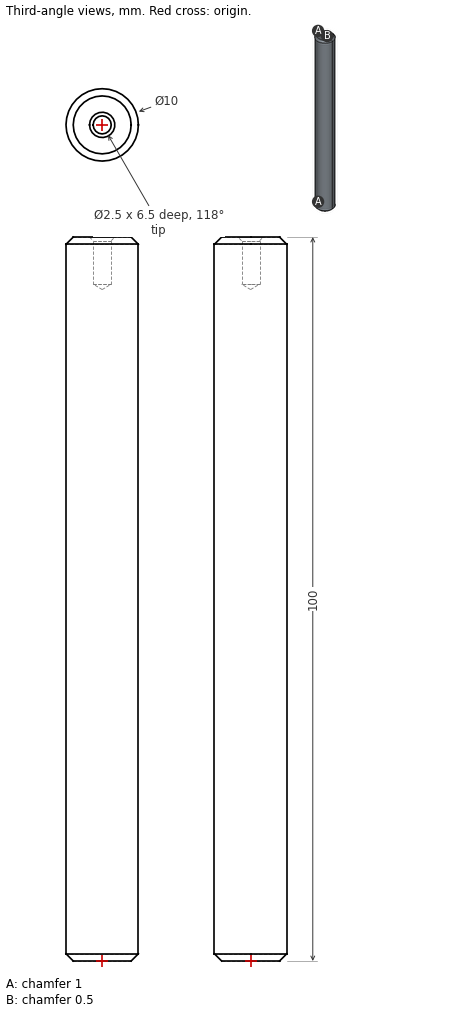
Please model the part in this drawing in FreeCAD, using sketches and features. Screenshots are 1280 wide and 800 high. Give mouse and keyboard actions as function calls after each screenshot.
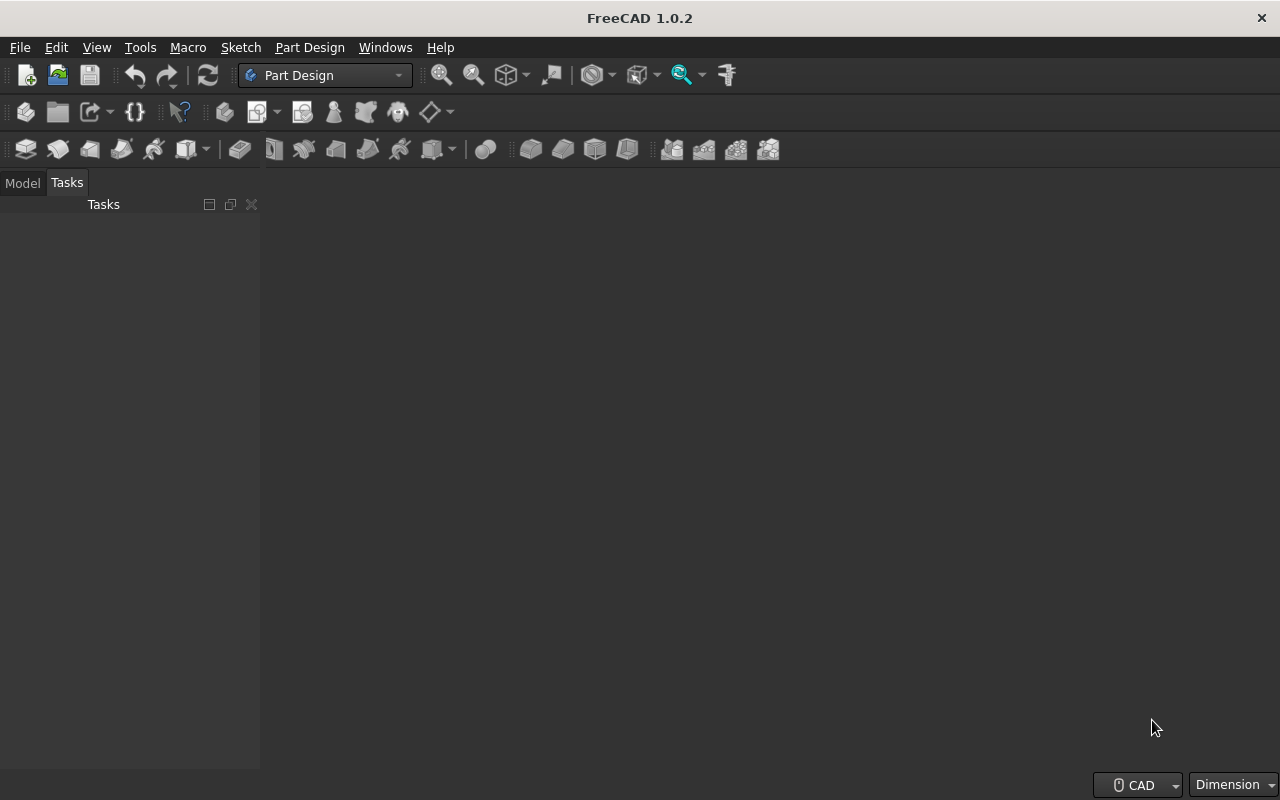
click(168, 112)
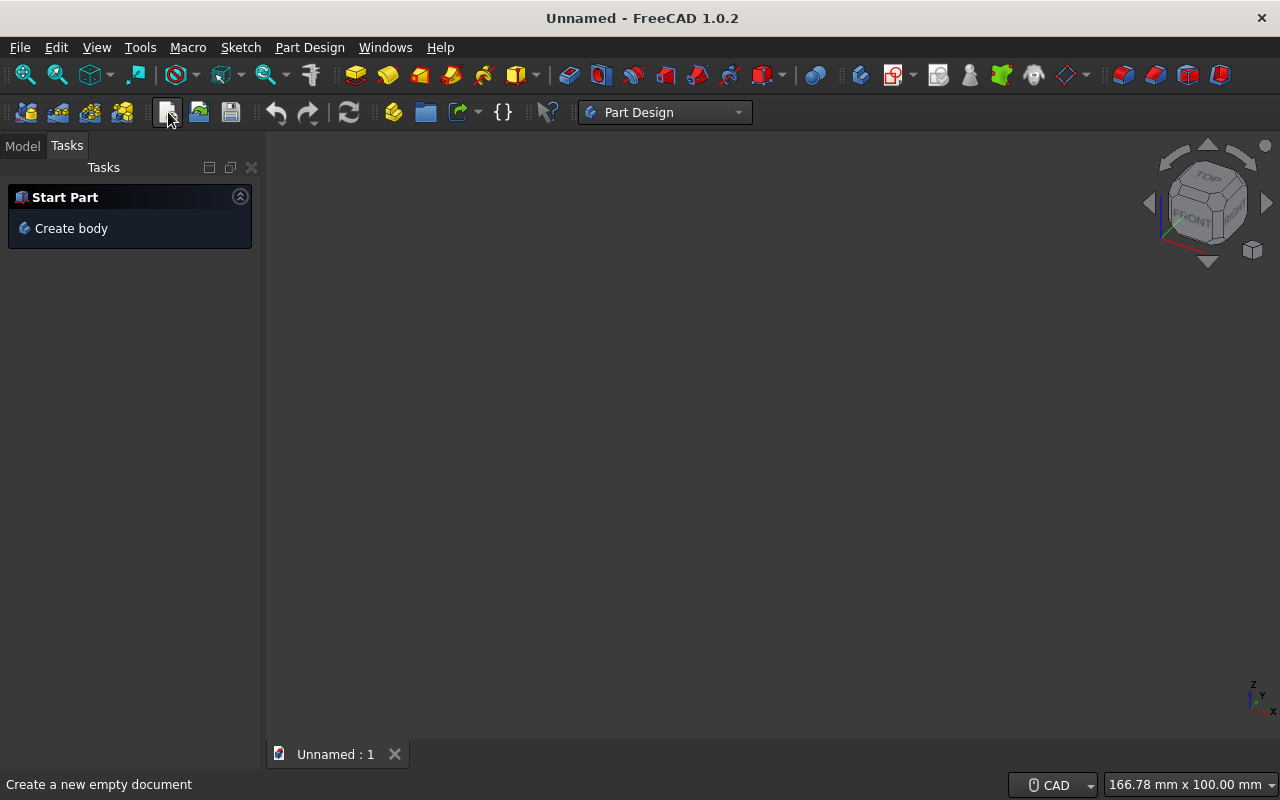
click(894, 76)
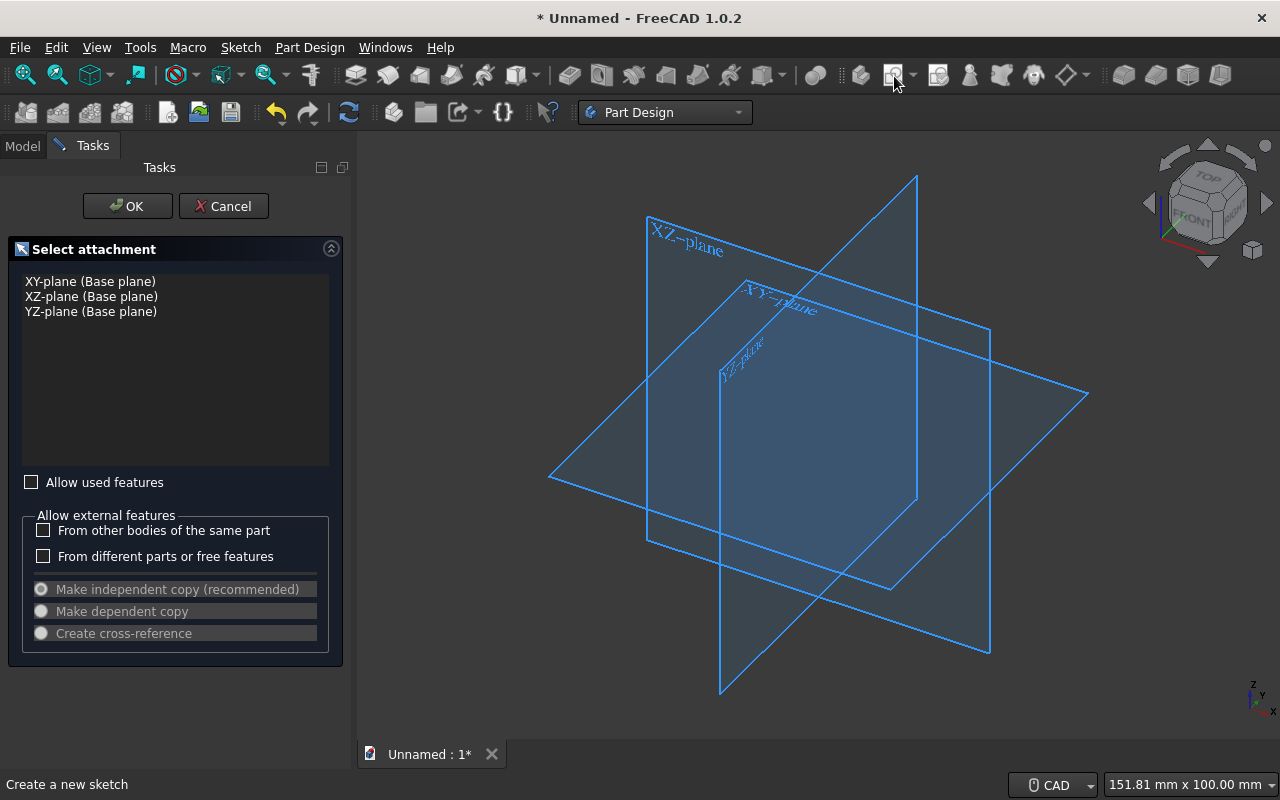
click(82, 282)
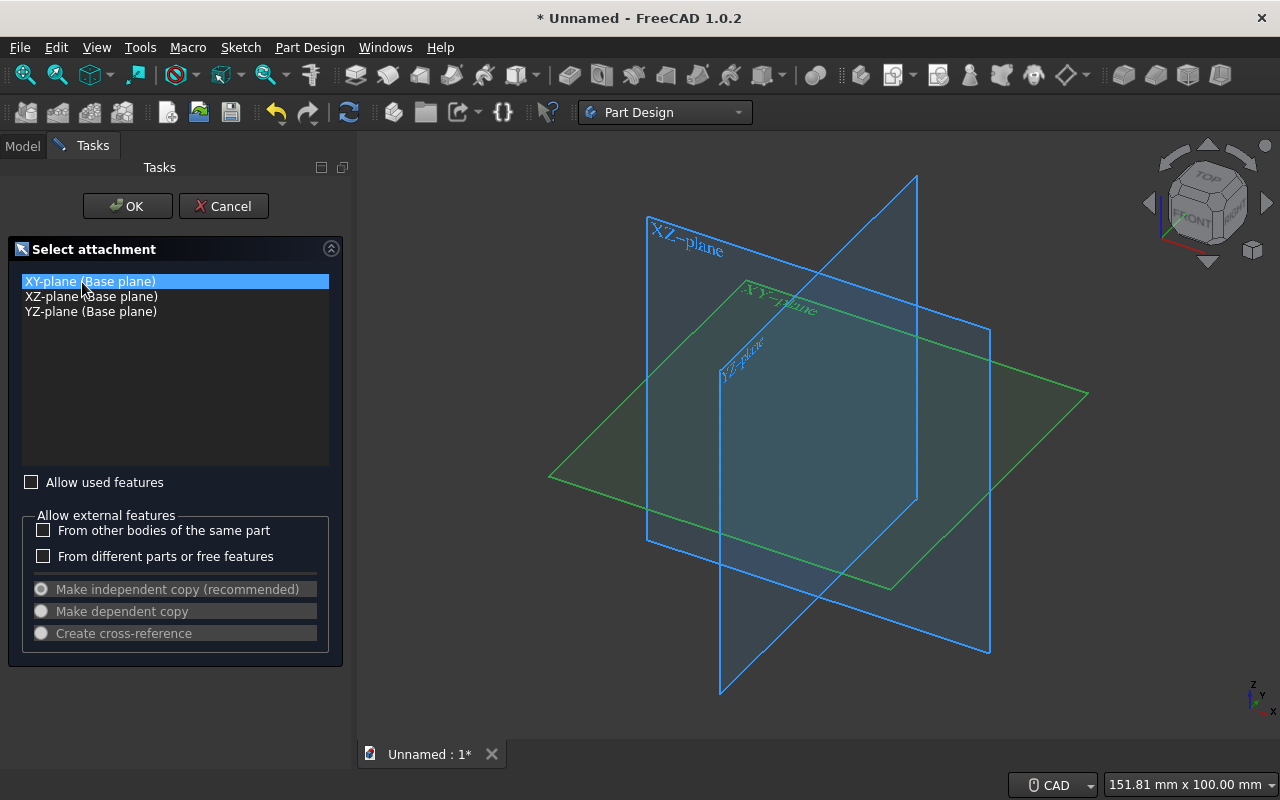
click(128, 206)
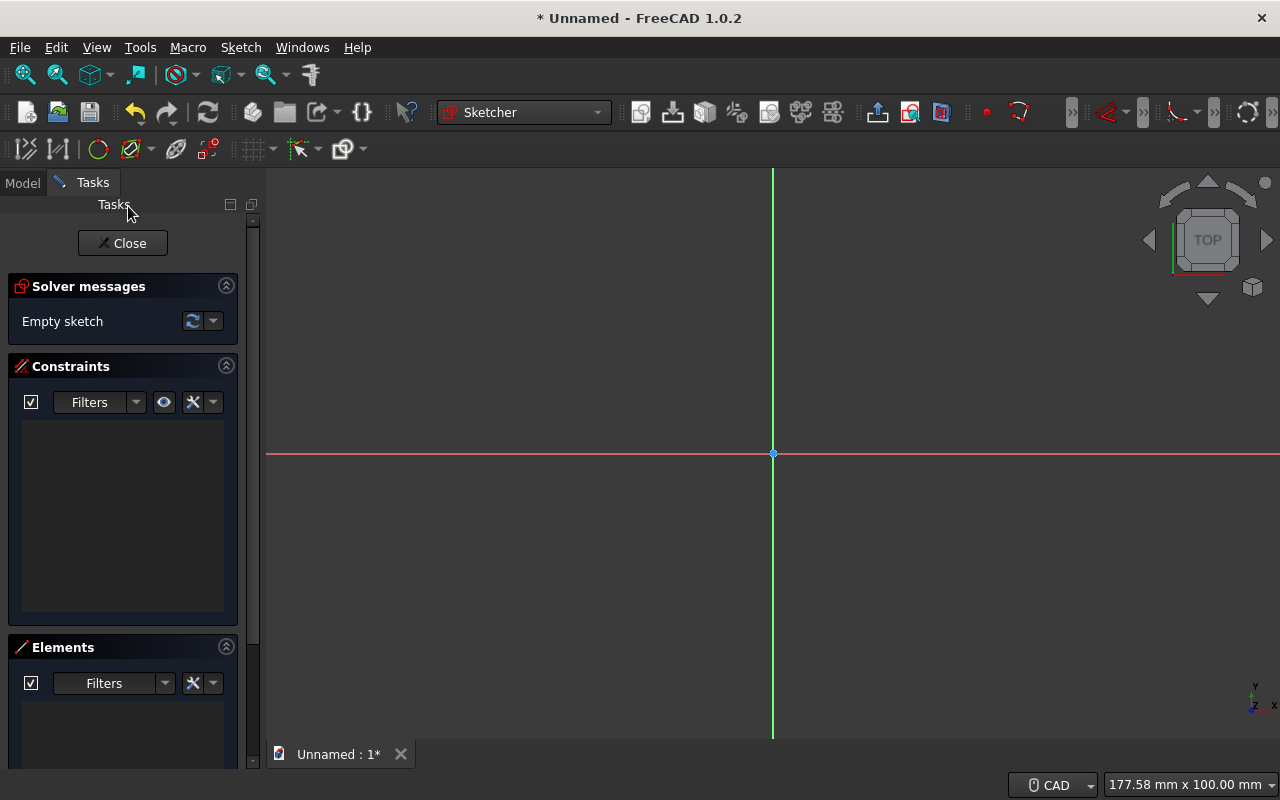
scroll(787, 454, up, 9)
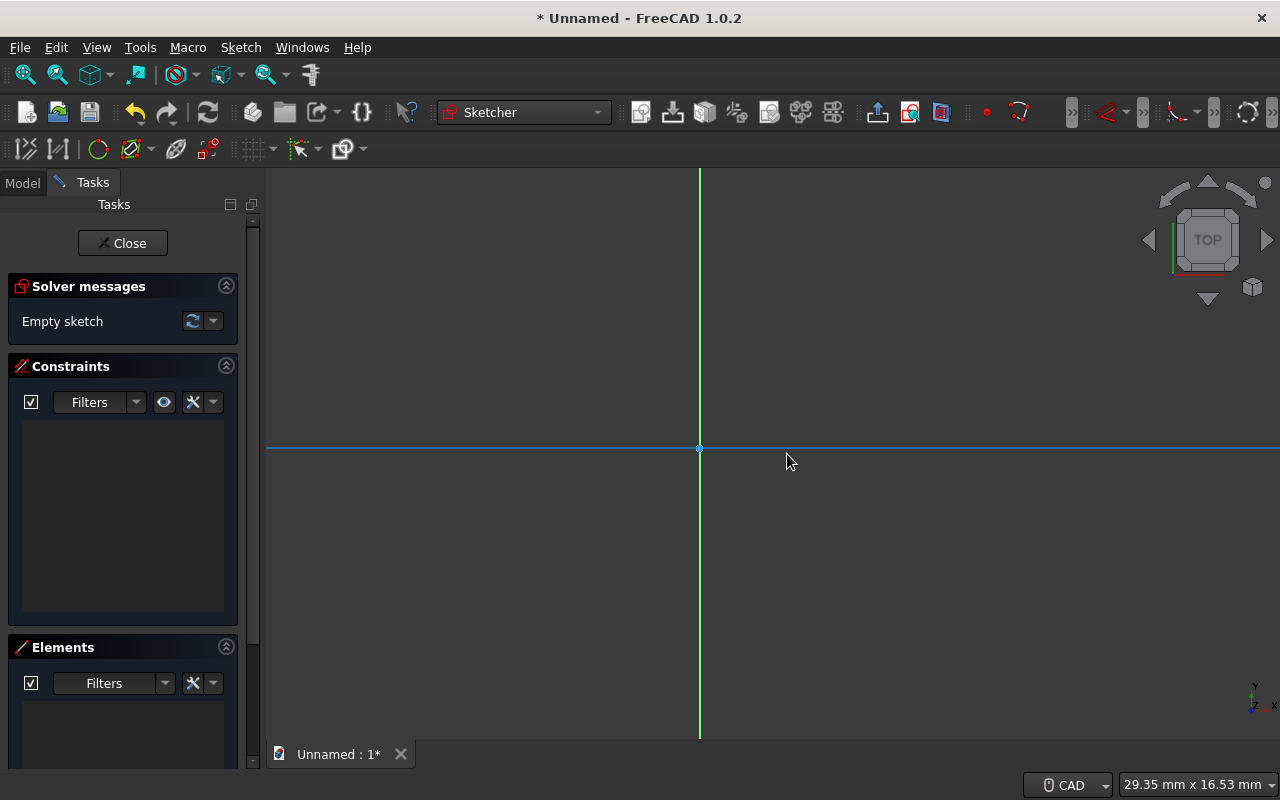
key(g)
key(c)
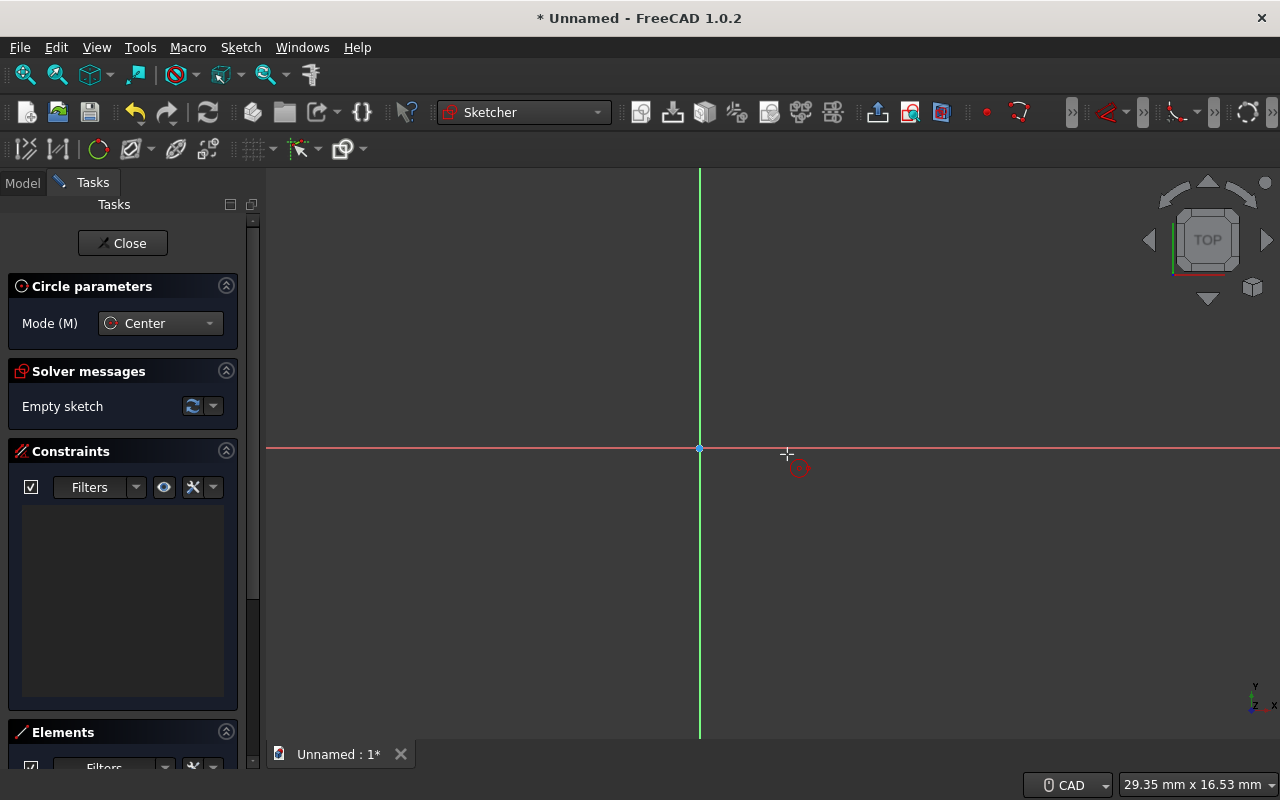
click(700, 448)
move(822, 326)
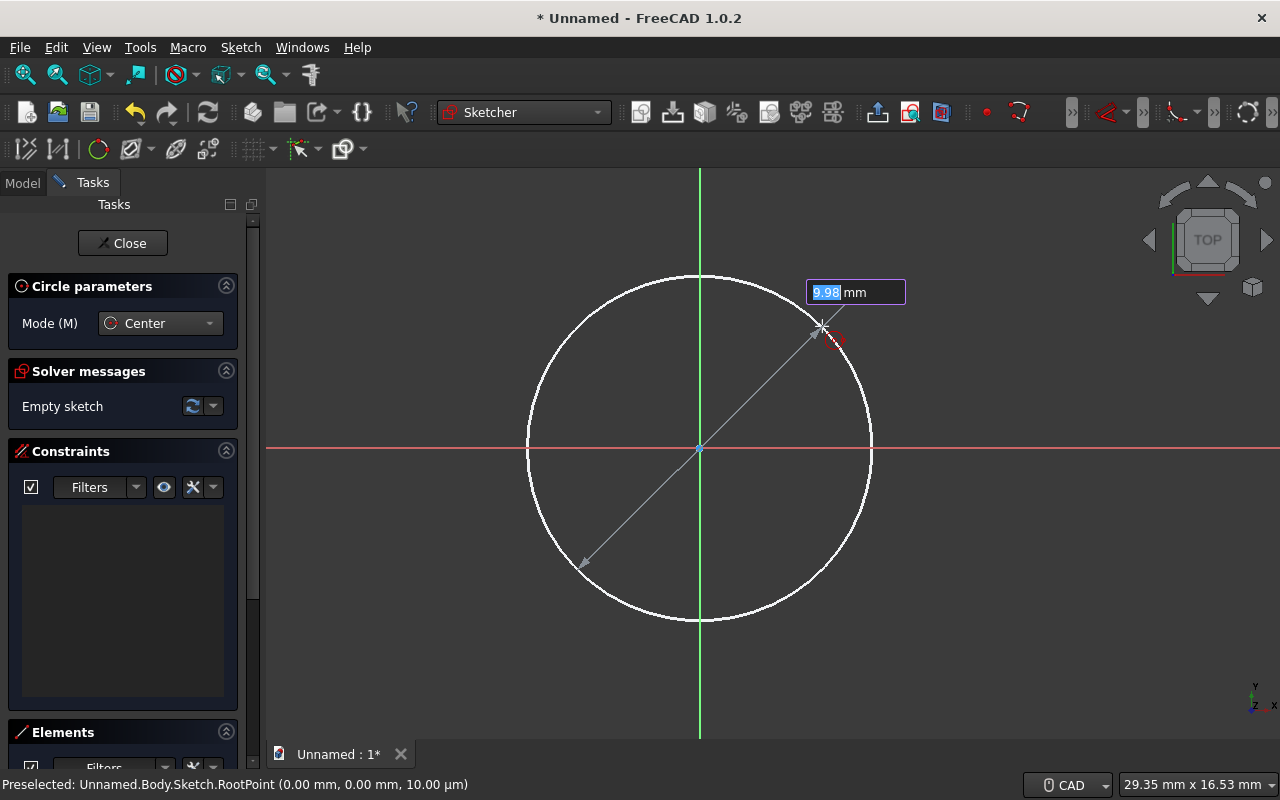
text(10)
key(Return)
key(Escape)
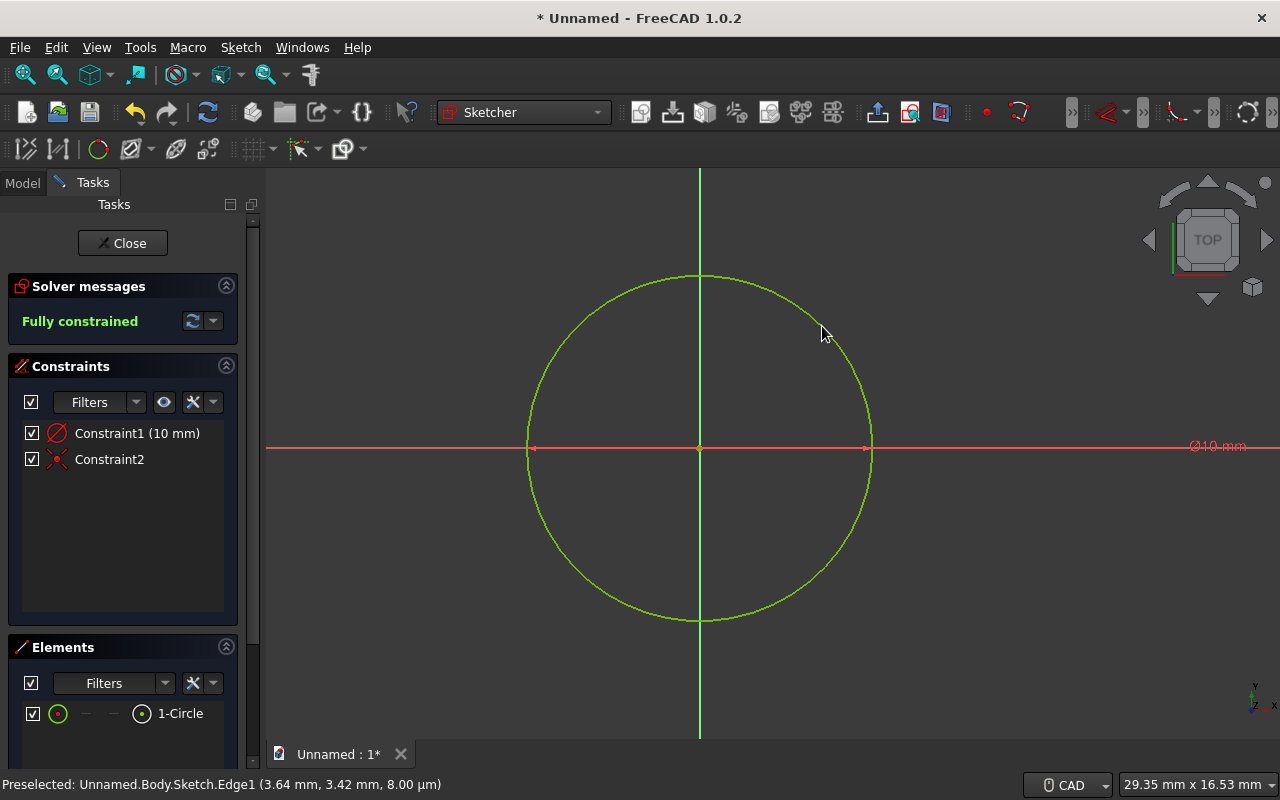
click(123, 243)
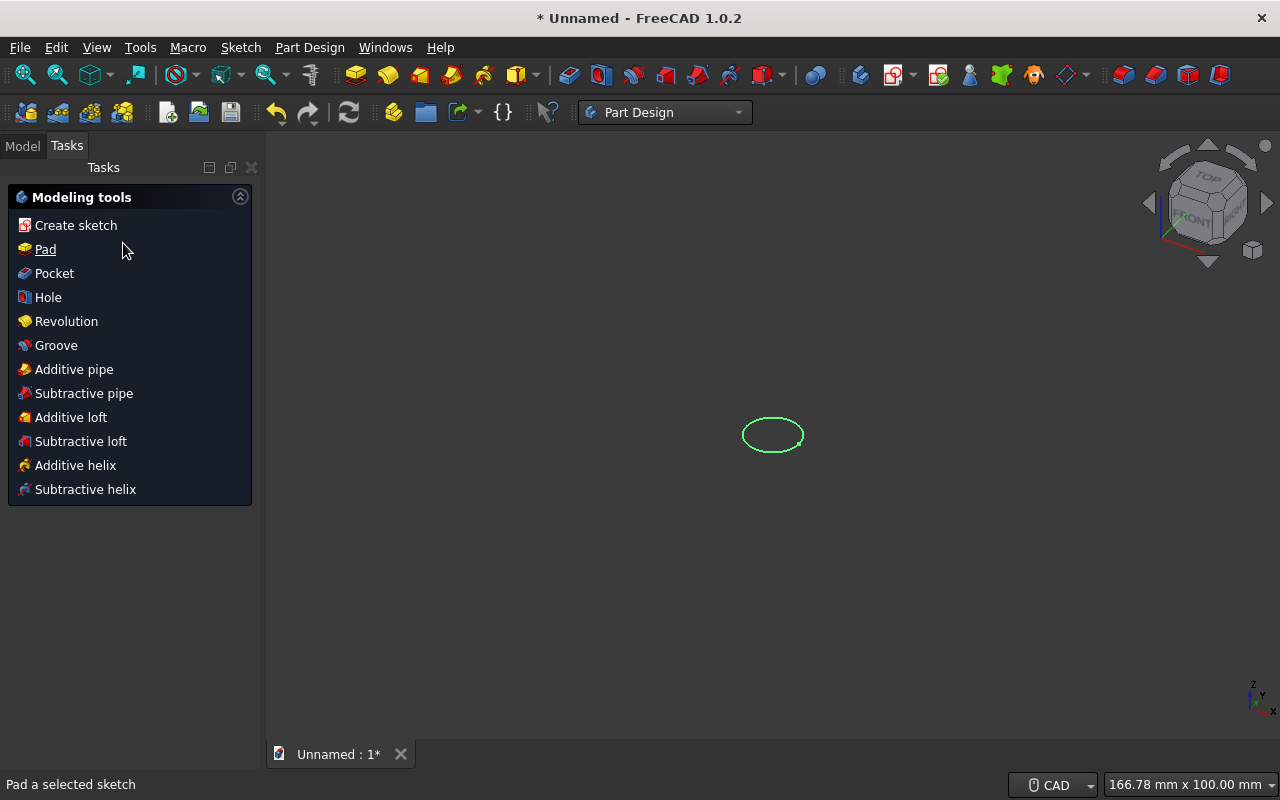
click(356, 76)